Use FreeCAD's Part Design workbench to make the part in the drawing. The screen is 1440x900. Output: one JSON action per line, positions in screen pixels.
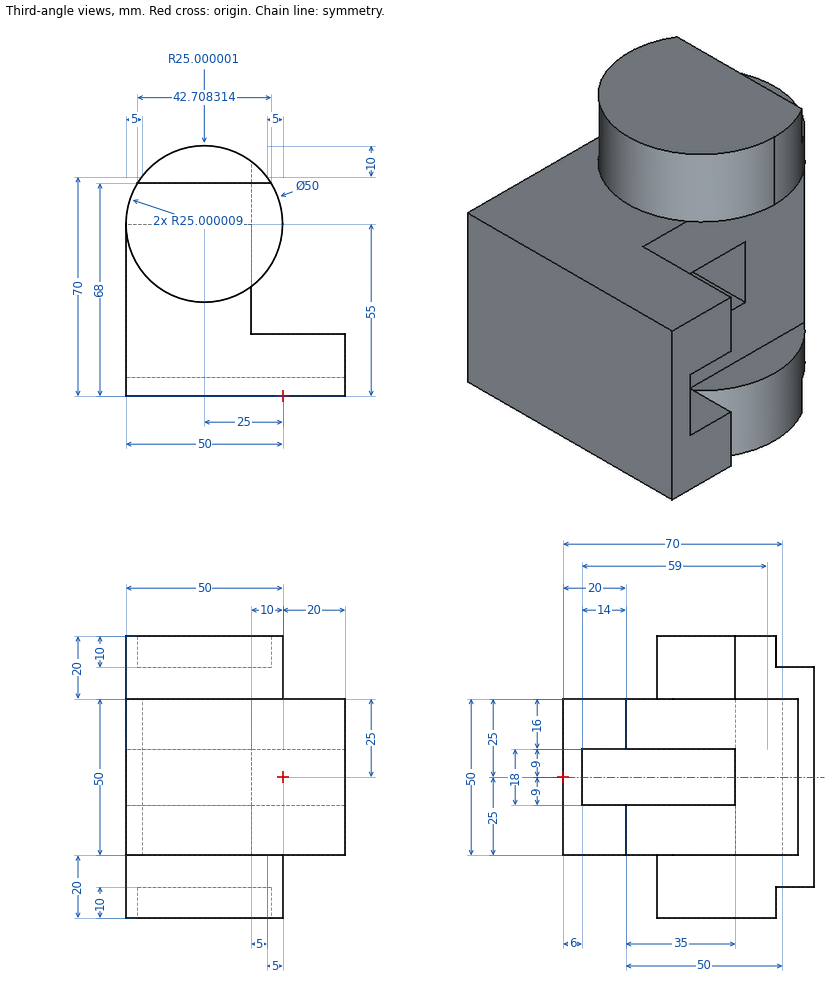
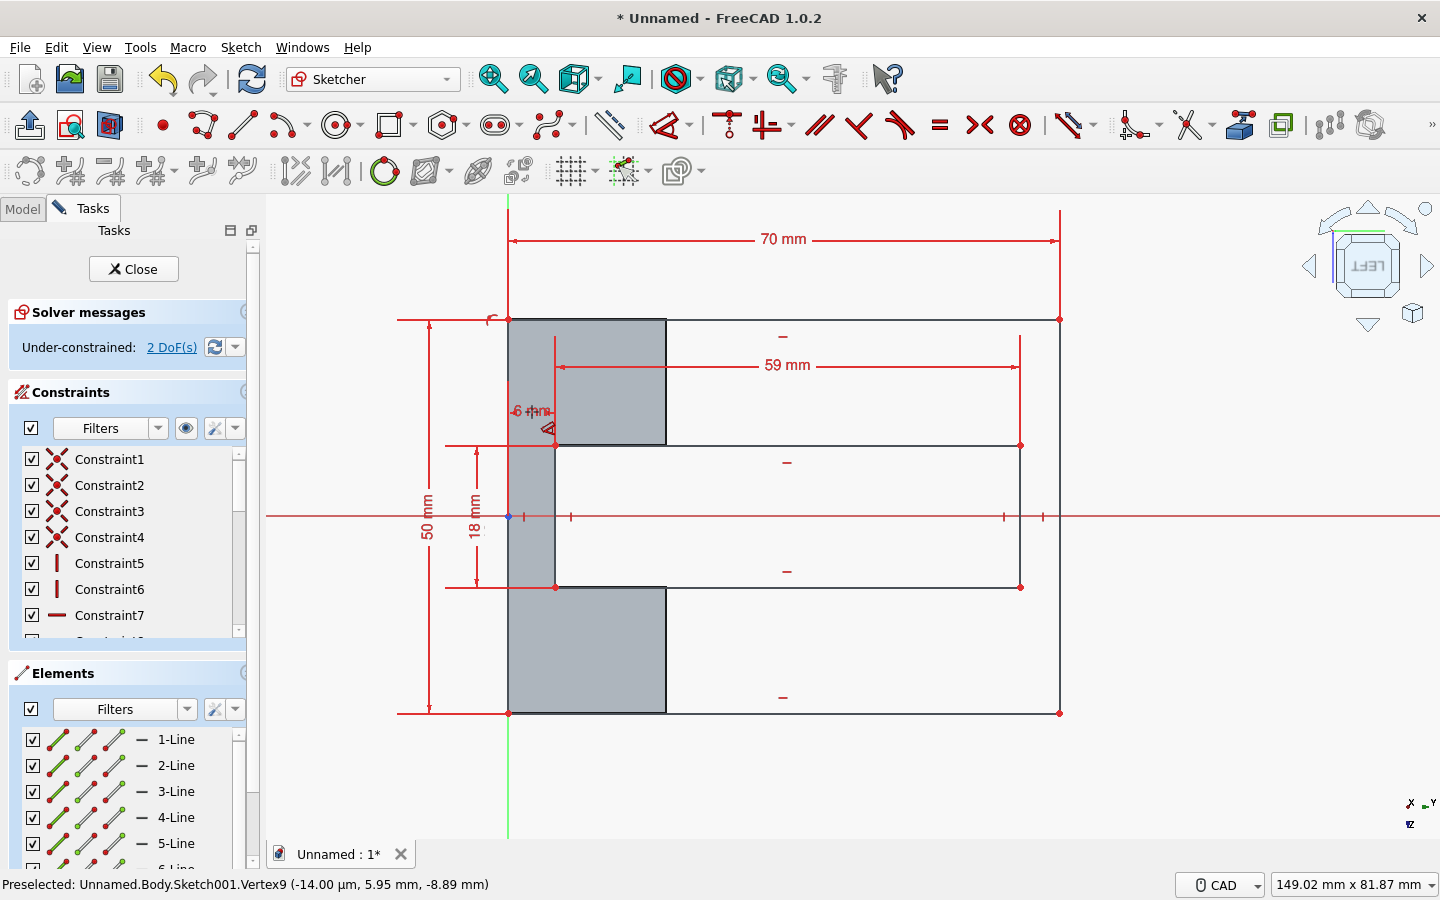
{"action": "left_click", "coordinate": [555, 446]}
{"action": "left_click", "coordinate": [474, 481]}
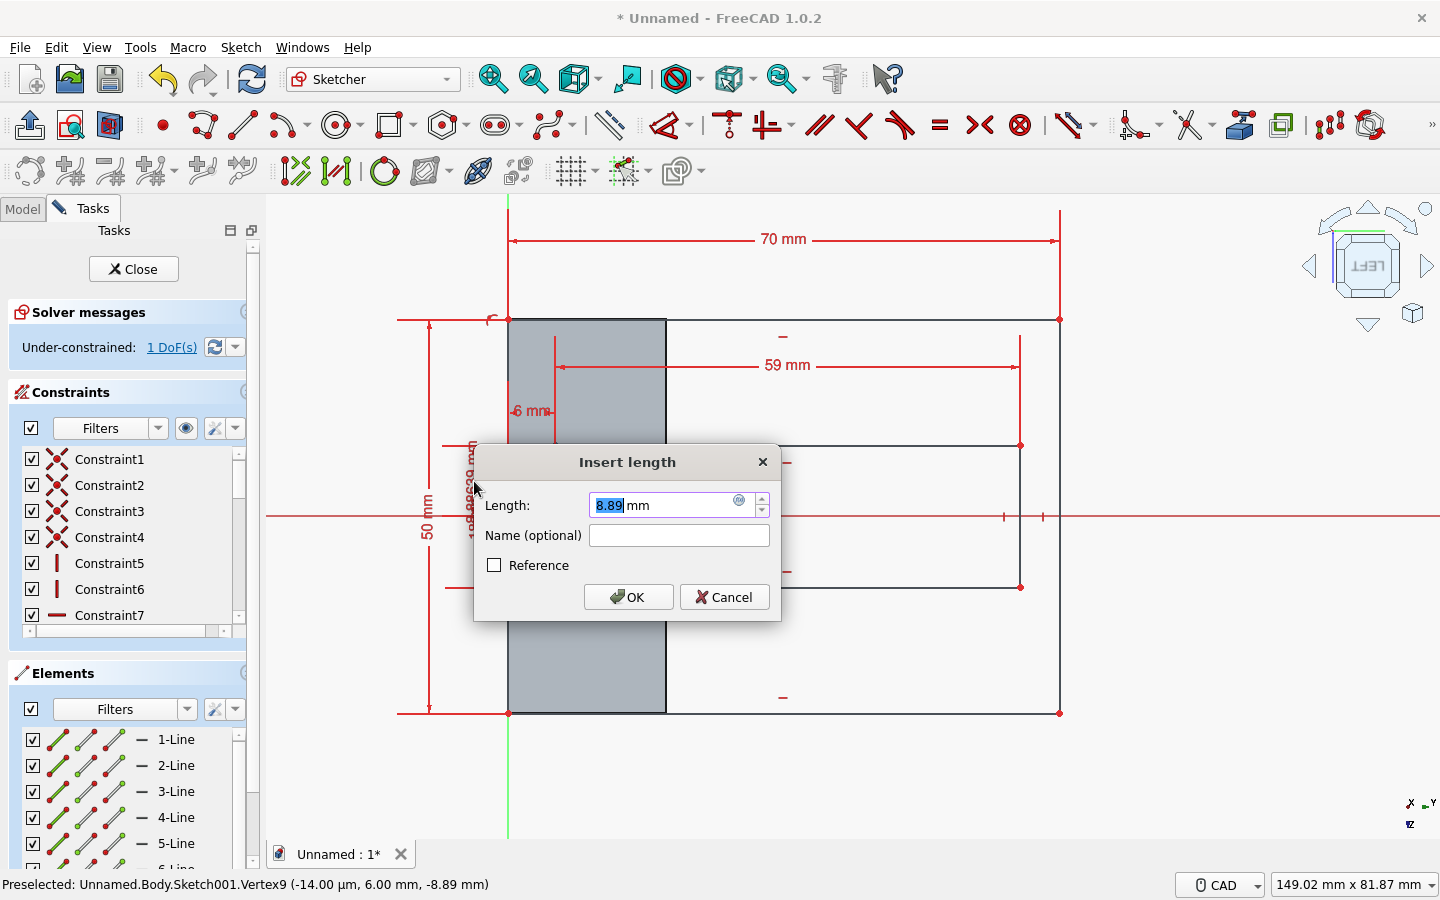
{"action": "type", "text": "9"}
{"action": "key", "text": "Return"}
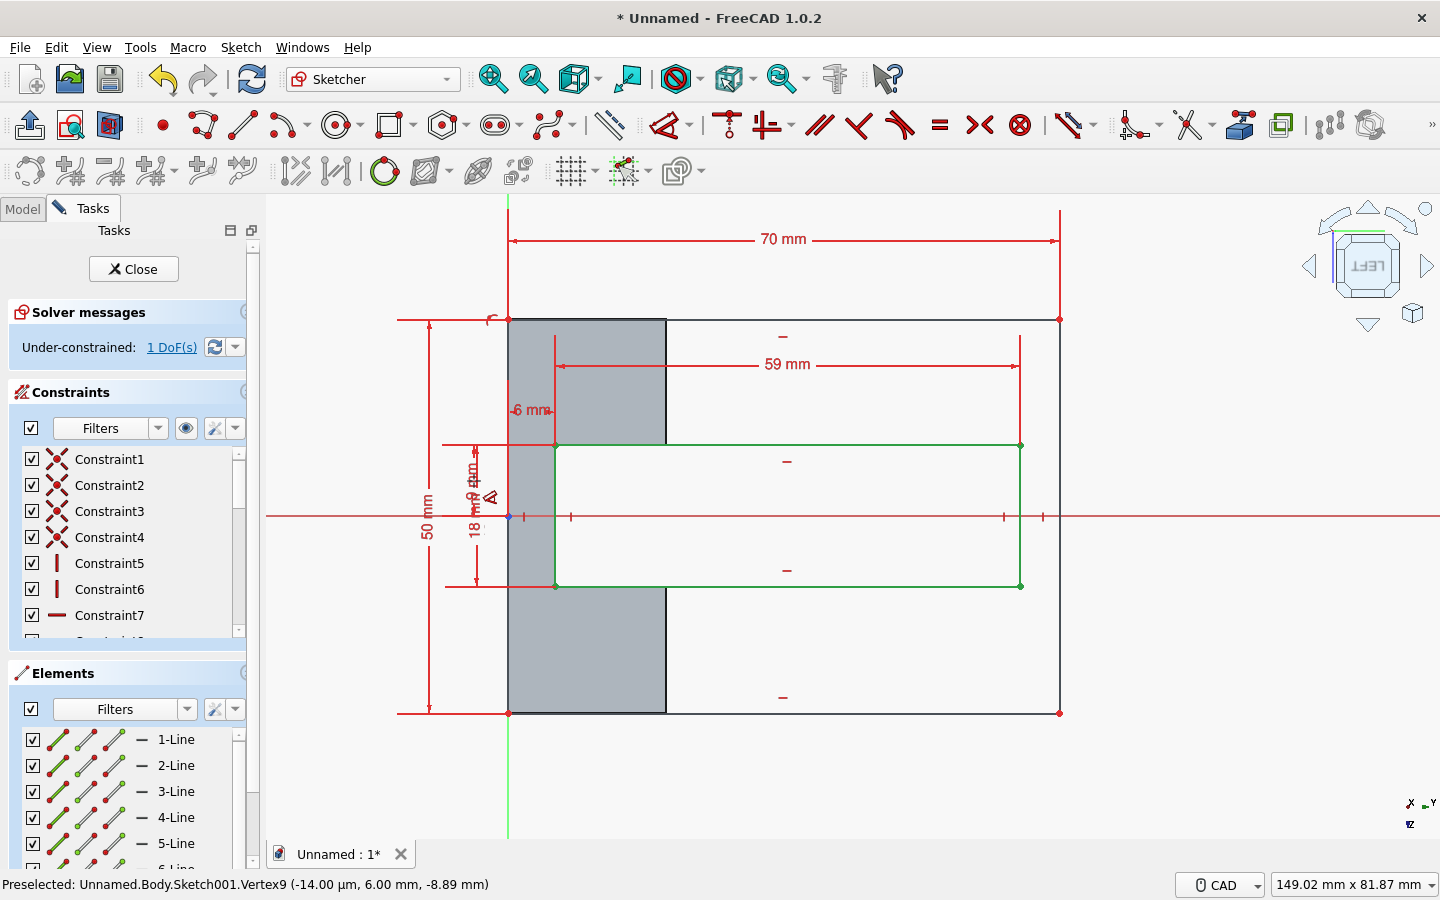
{"action": "left_click", "coordinate": [508, 320]}
{"action": "left_click", "coordinate": [474, 373]}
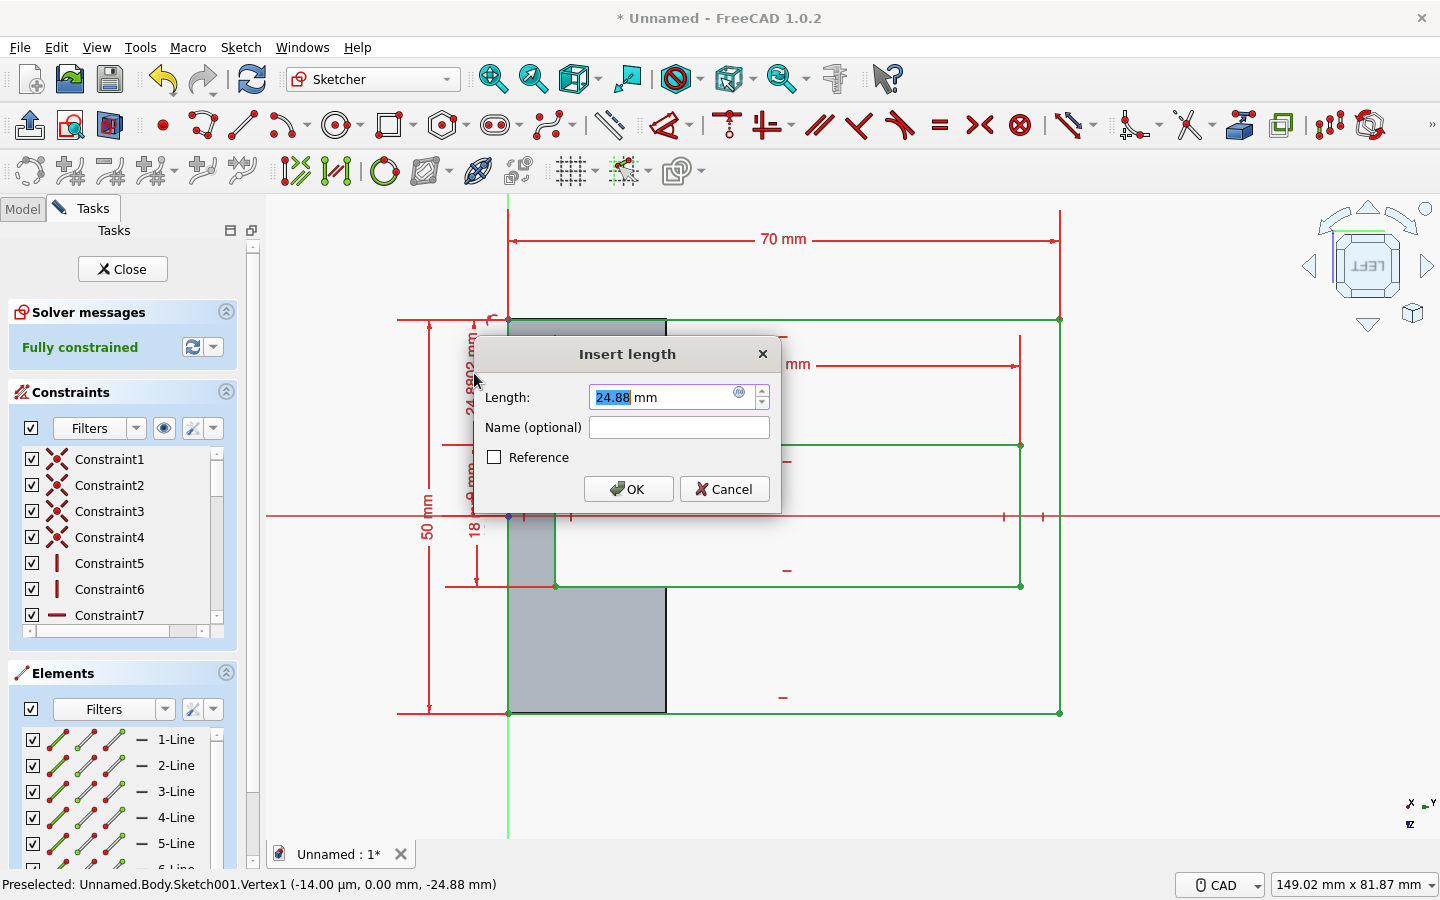
{"action": "type", "text": "25"}
{"action": "key", "text": "Return"}
{"action": "key", "text": "Escape"}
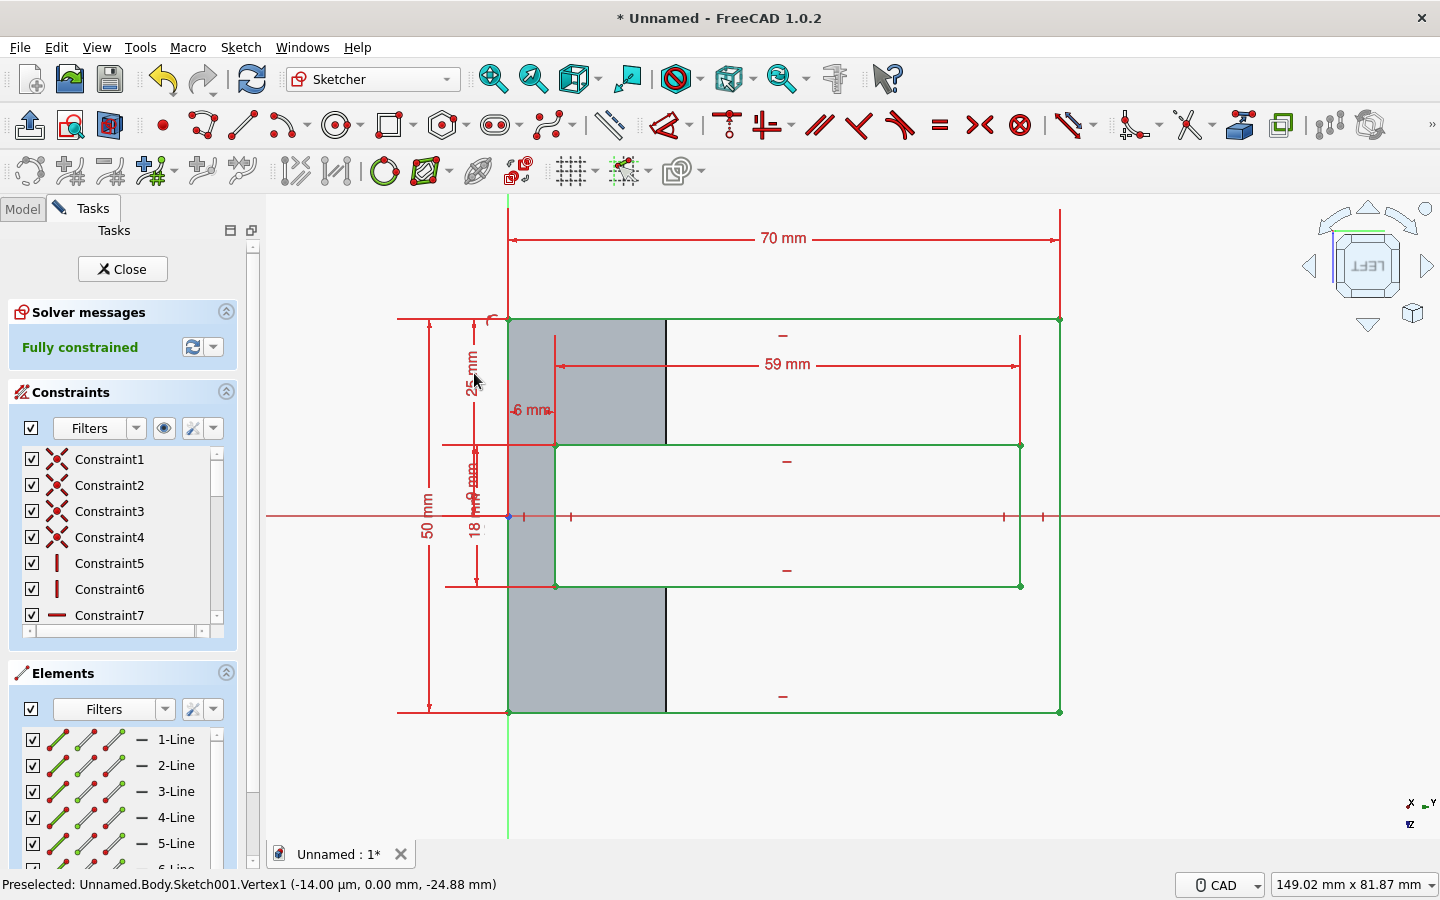
{"action": "left_click", "coordinate": [123, 269]}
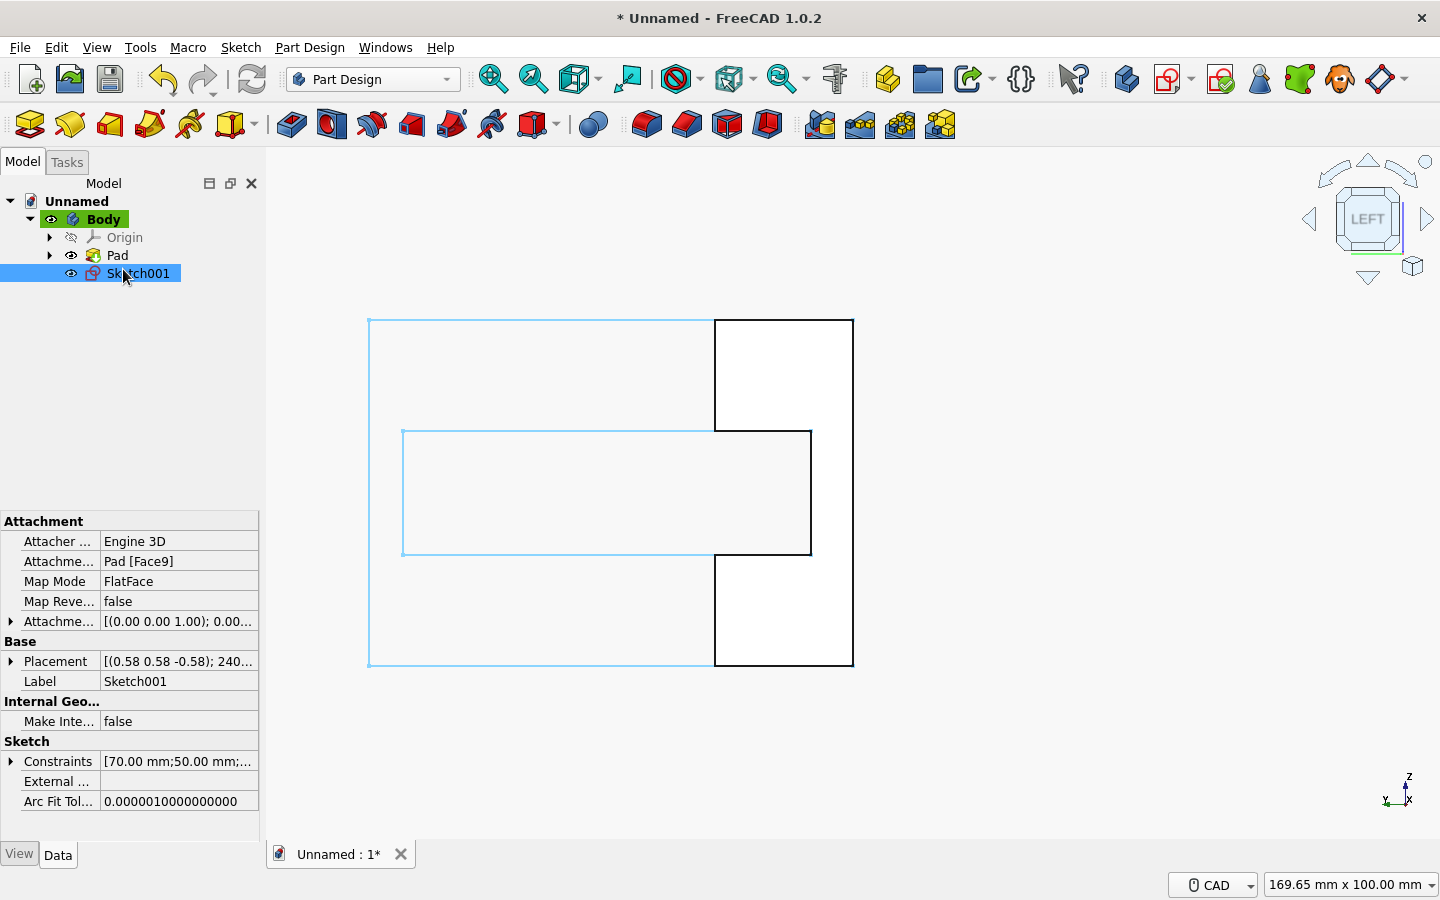
{"action": "left_click", "coordinate": [30, 124]}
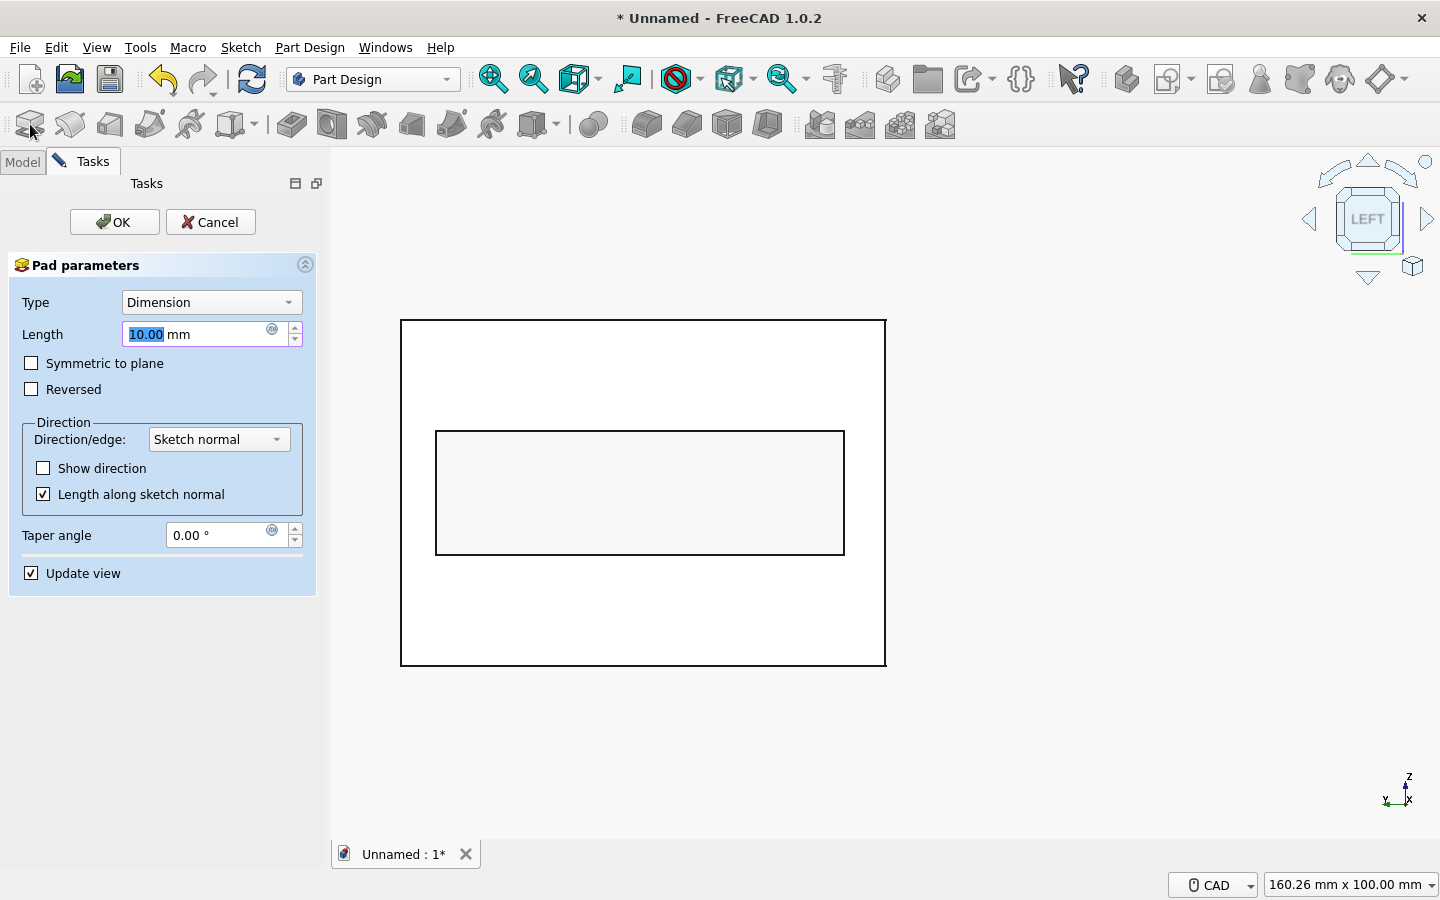
{"action": "type", "text": "50"}
{"action": "key", "text": "Tab"}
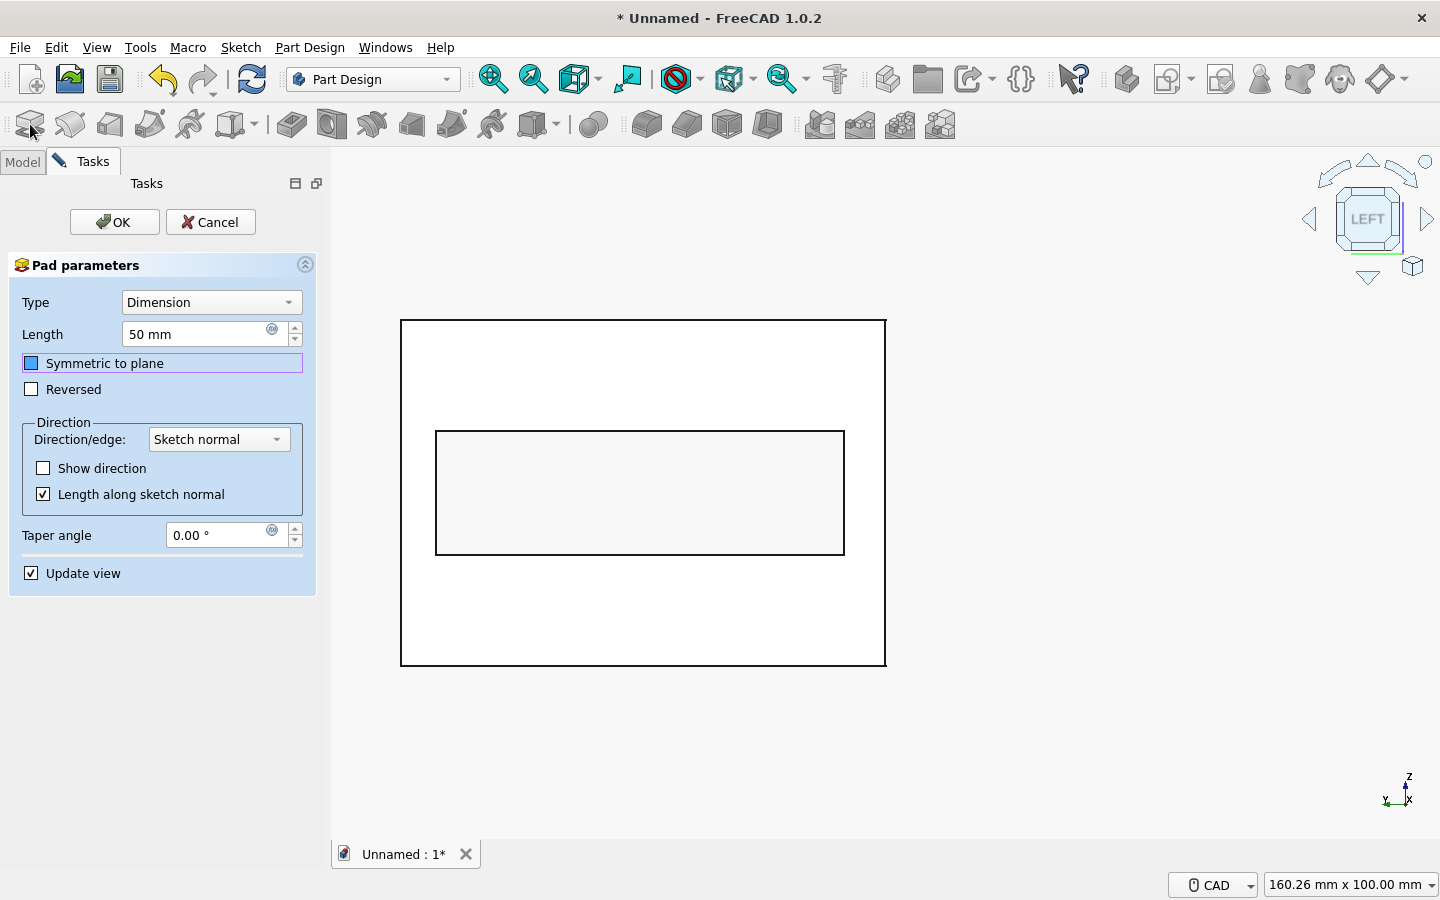
{"action": "left_click", "coordinate": [115, 222]}